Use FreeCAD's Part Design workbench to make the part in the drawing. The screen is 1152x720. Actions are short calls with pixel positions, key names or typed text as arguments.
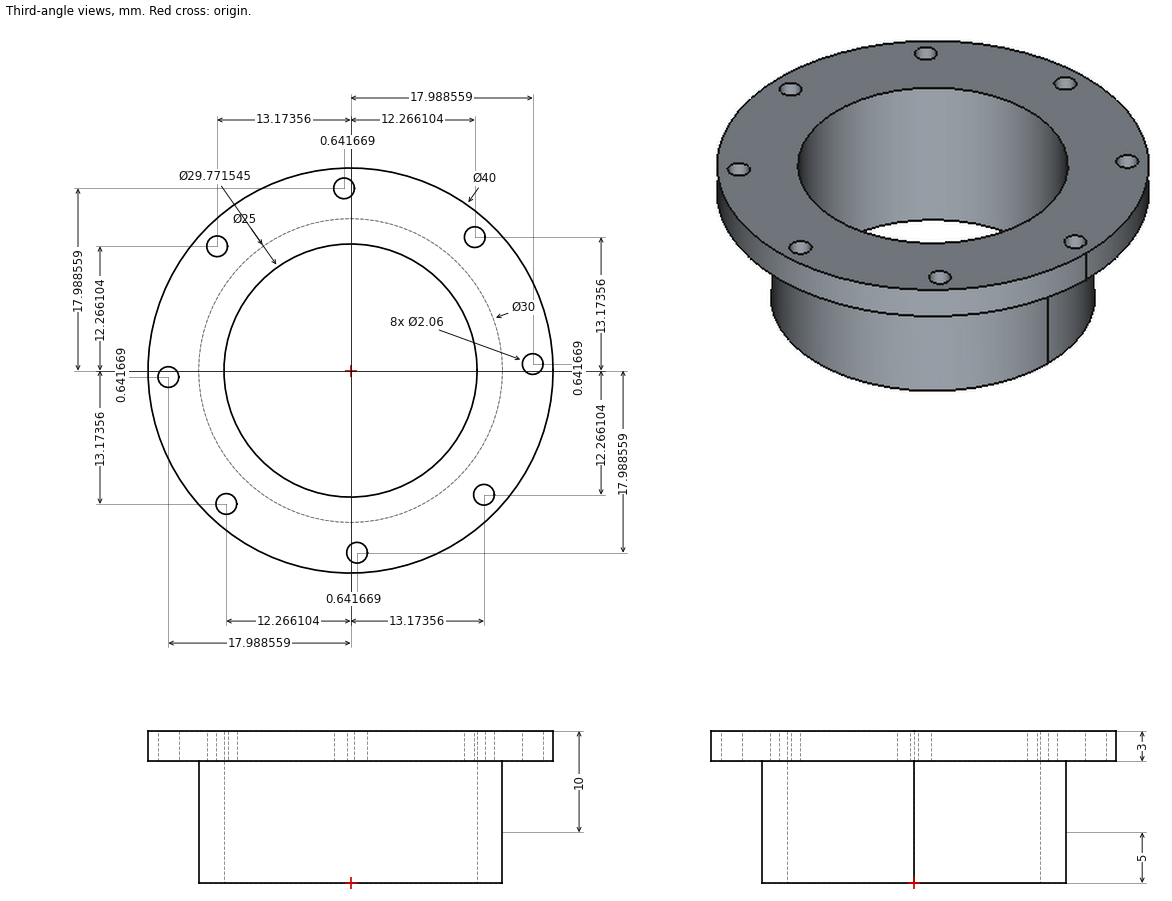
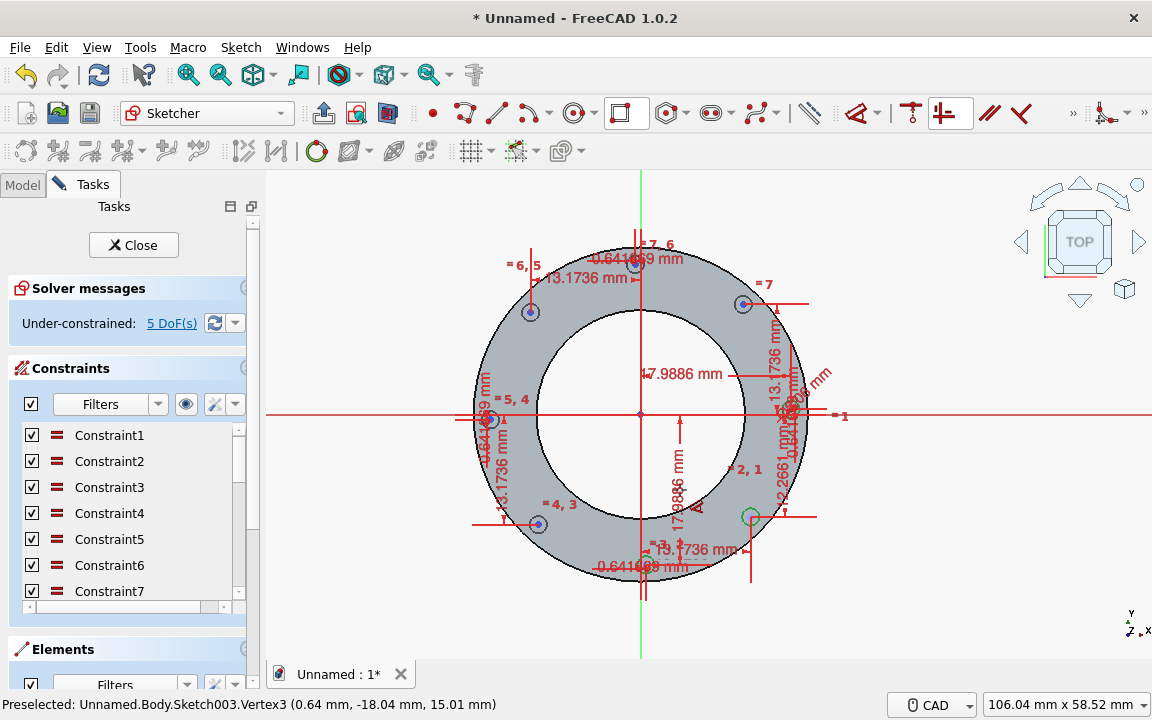
click(538, 525)
click(566, 559)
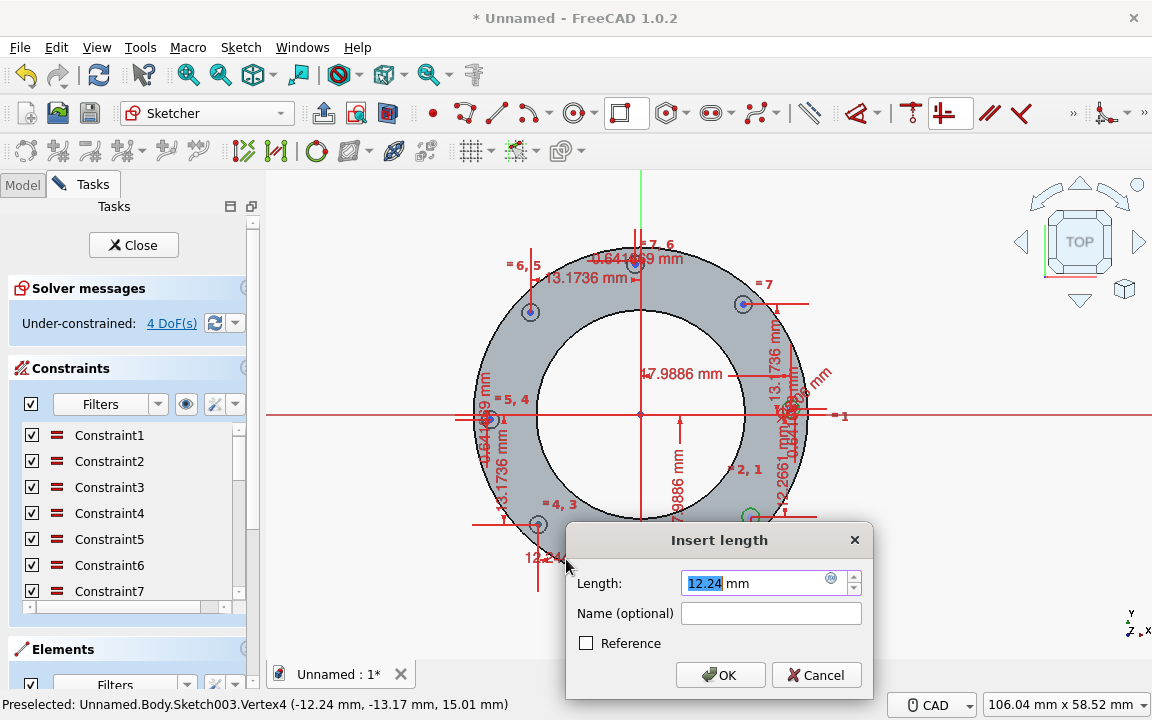
text(12.266104)
key(Return)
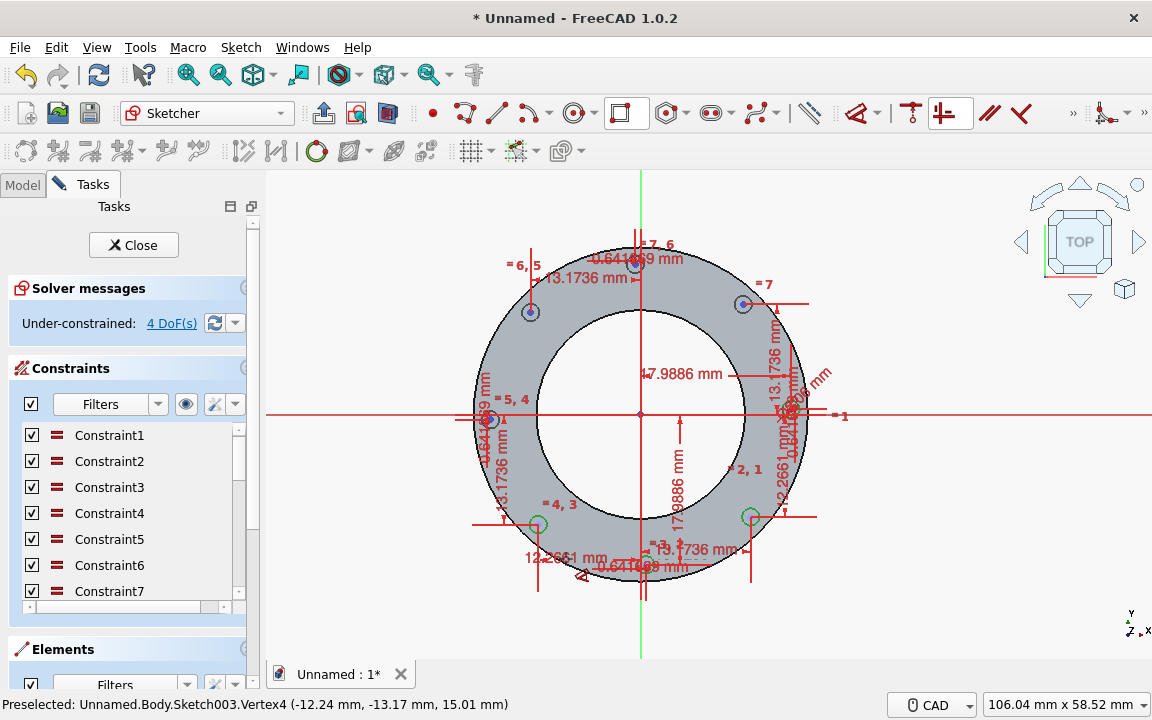
click(491, 420)
click(600, 454)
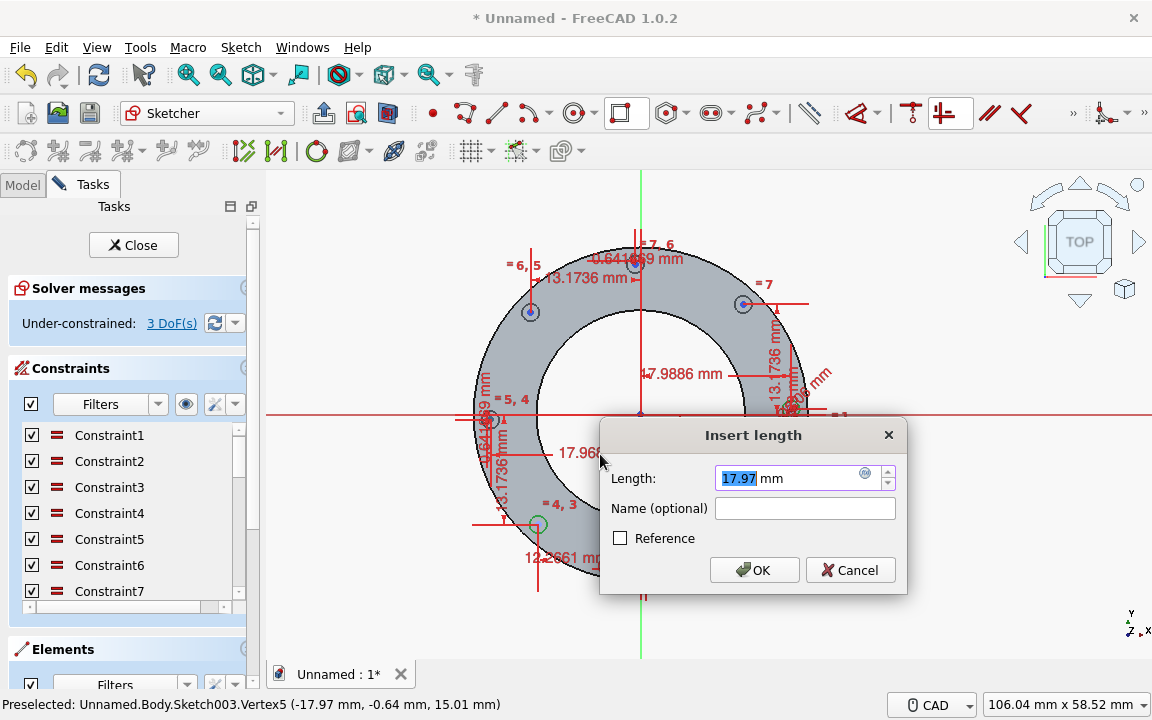
text(17.988559)
key(Return)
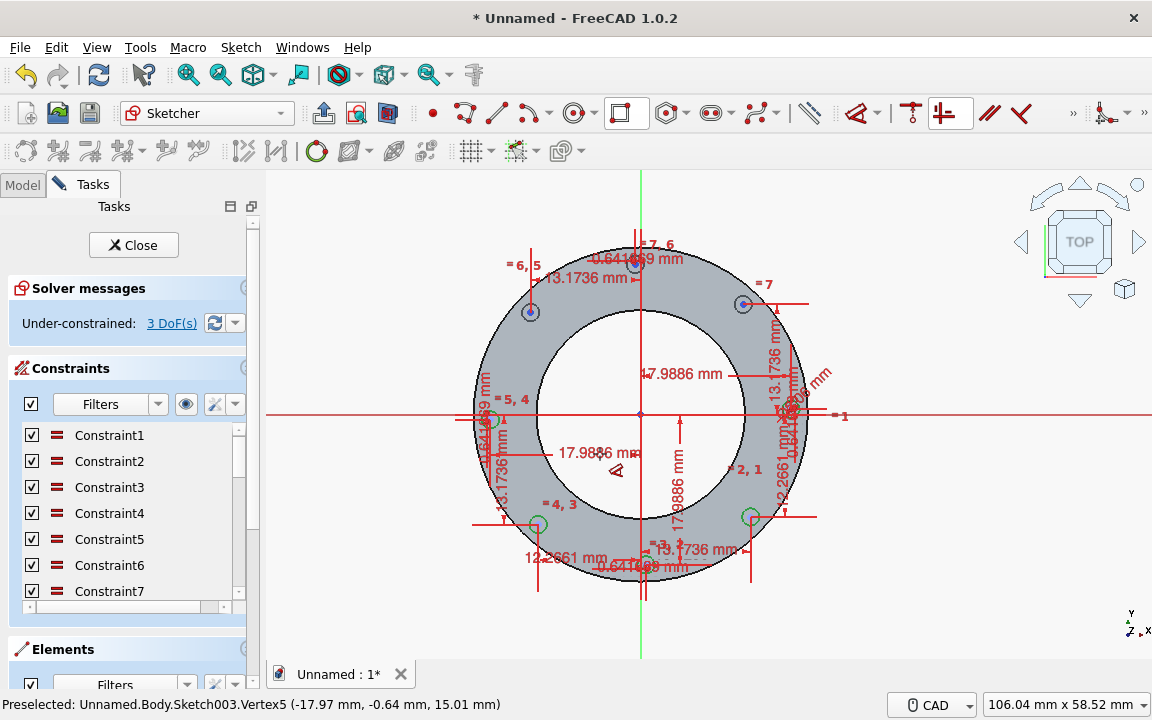
click(531, 313)
click(497, 364)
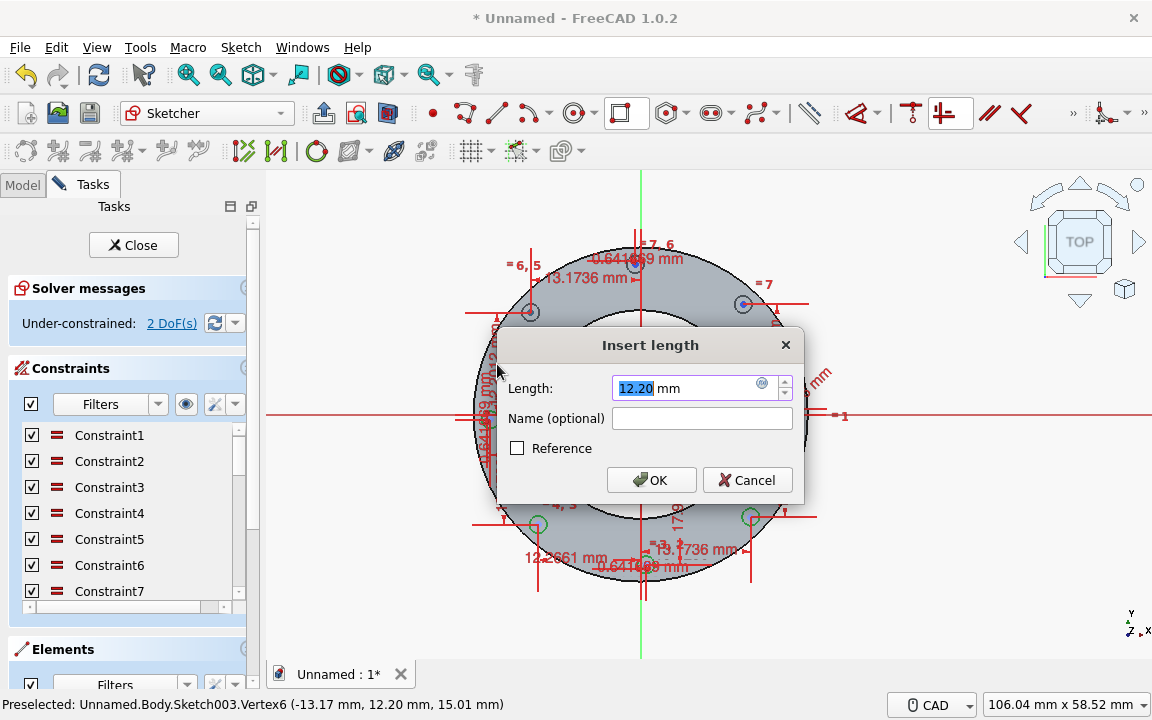
text(12.266104)
key(Return)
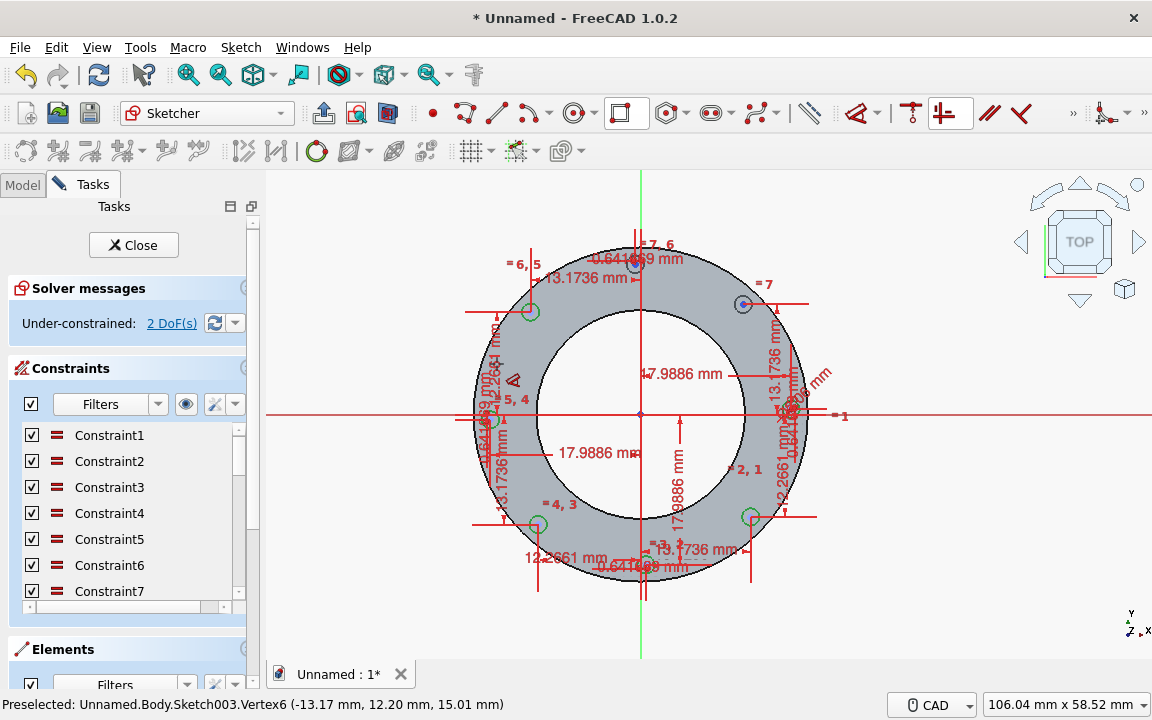
click(635, 264)
click(601, 340)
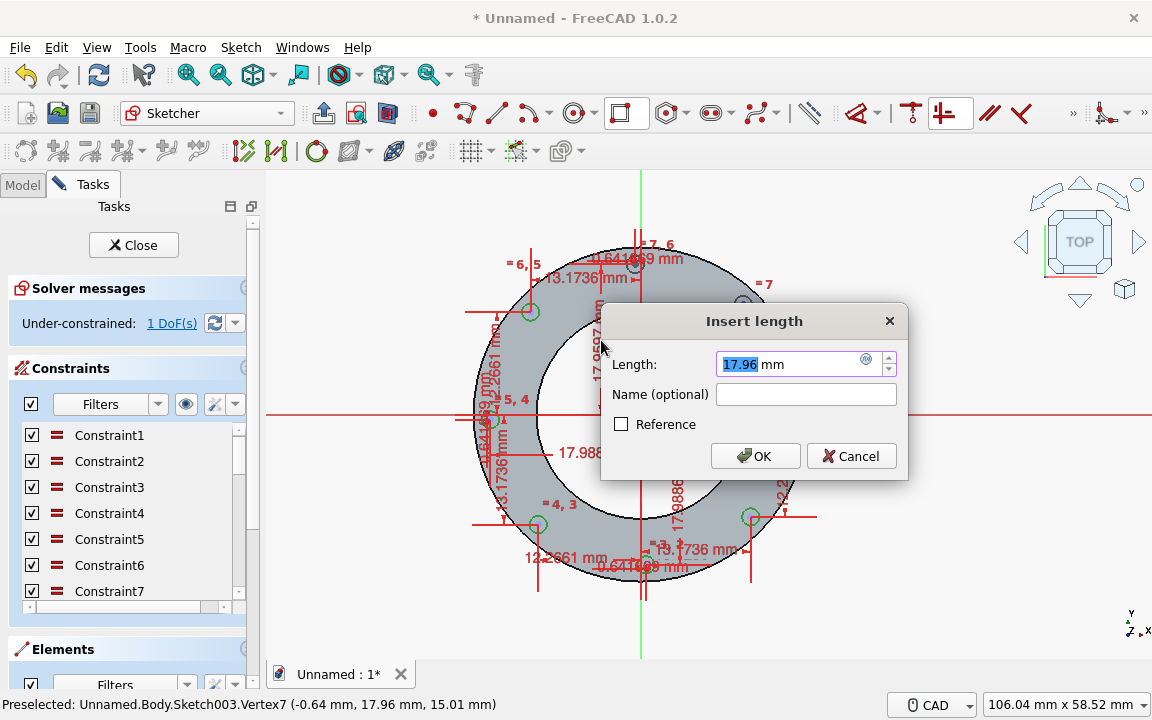
text(17.988559)
key(Return)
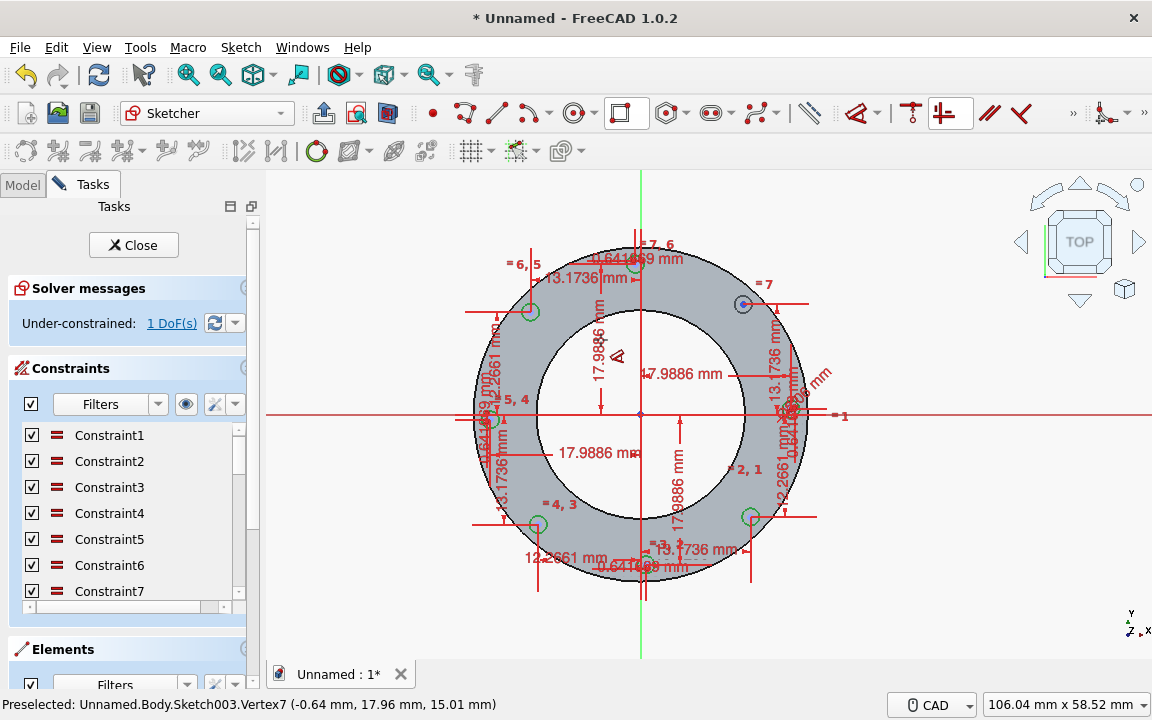
click(743, 304)
click(715, 270)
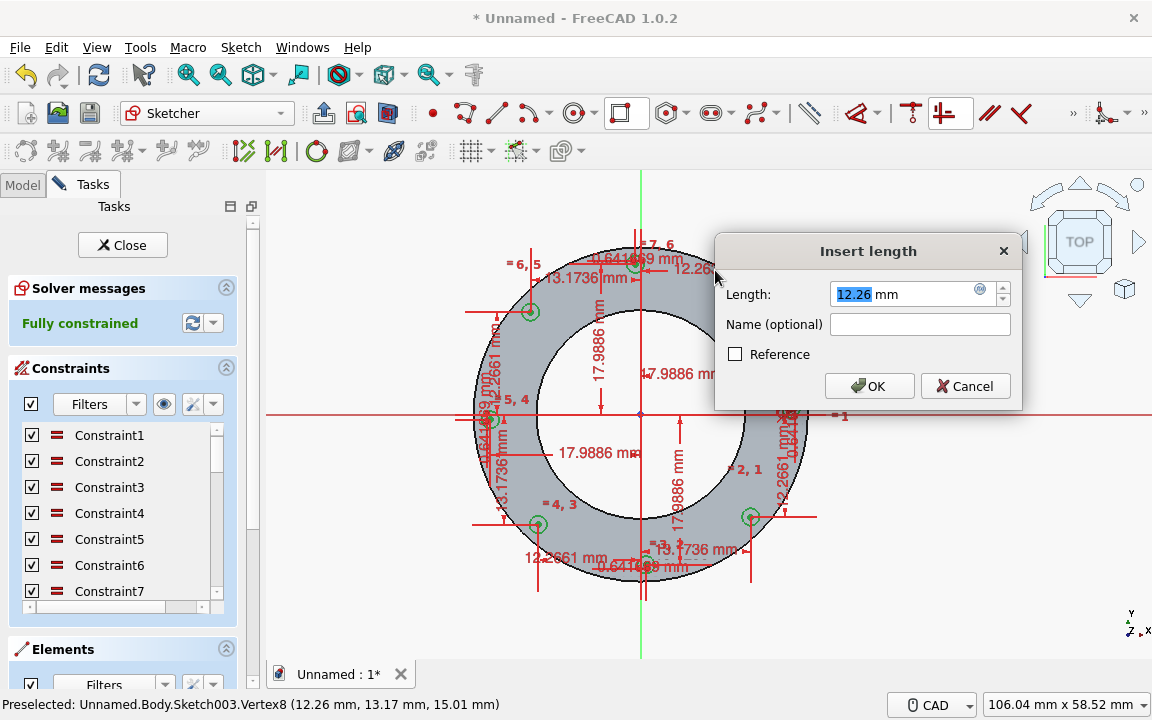
text(12.266104)
key(Return)
key(Escape)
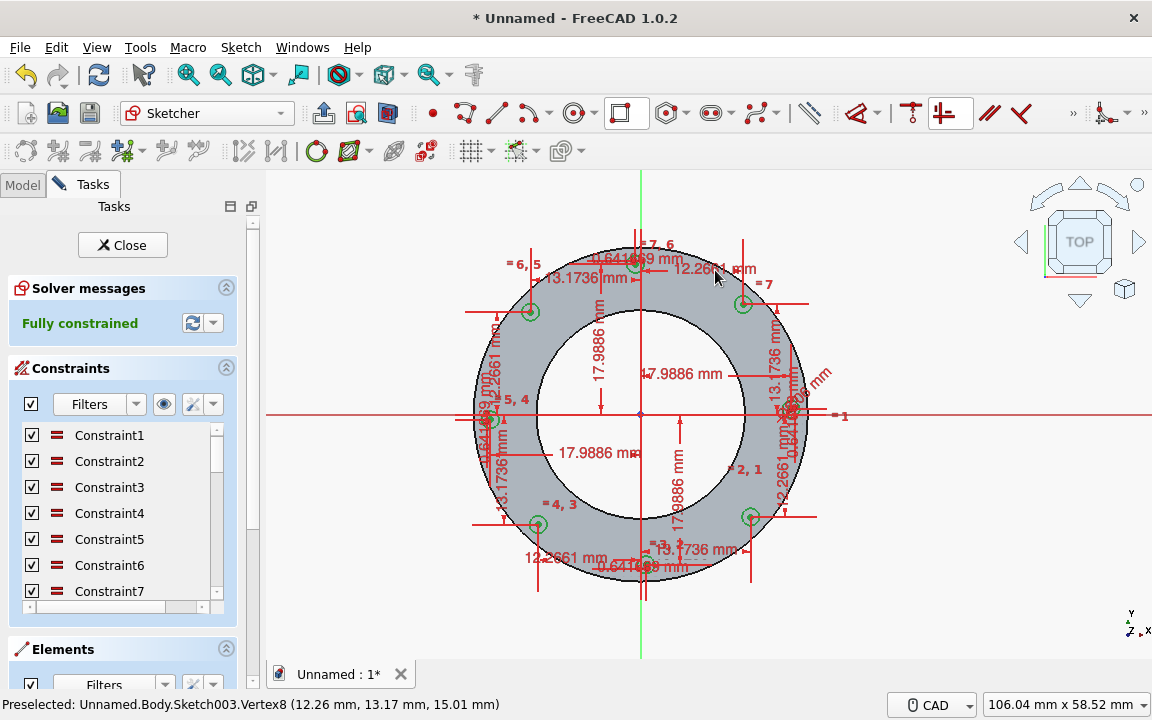
click(123, 245)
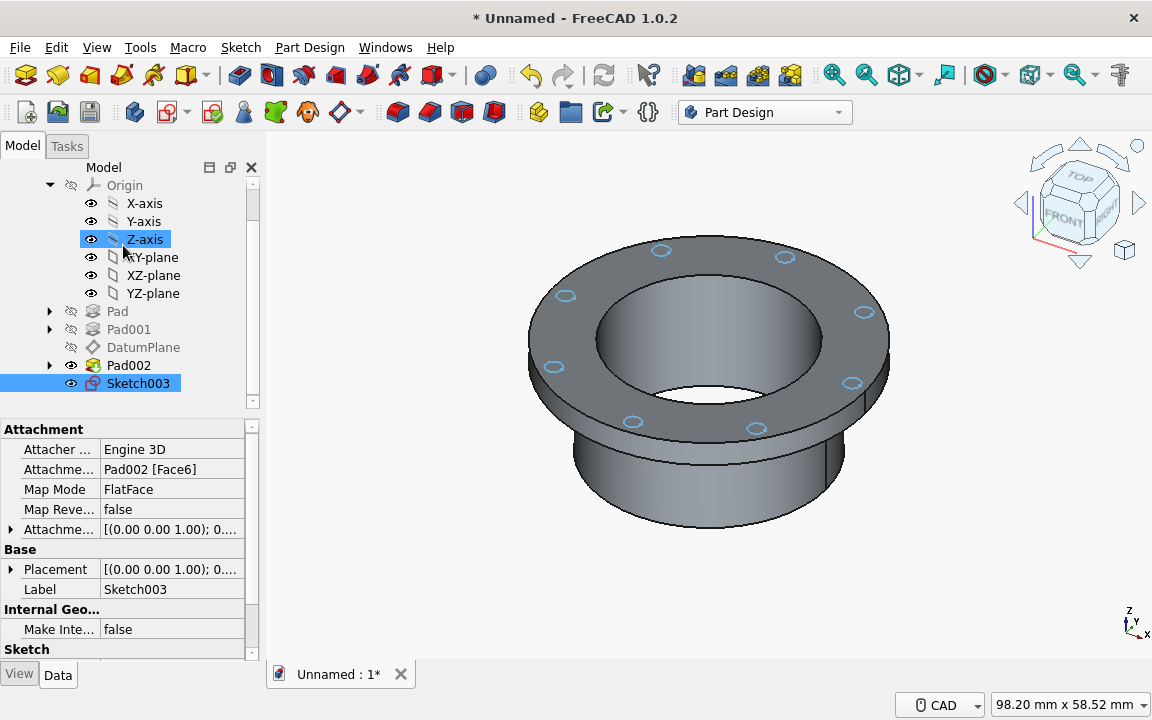
click(240, 76)